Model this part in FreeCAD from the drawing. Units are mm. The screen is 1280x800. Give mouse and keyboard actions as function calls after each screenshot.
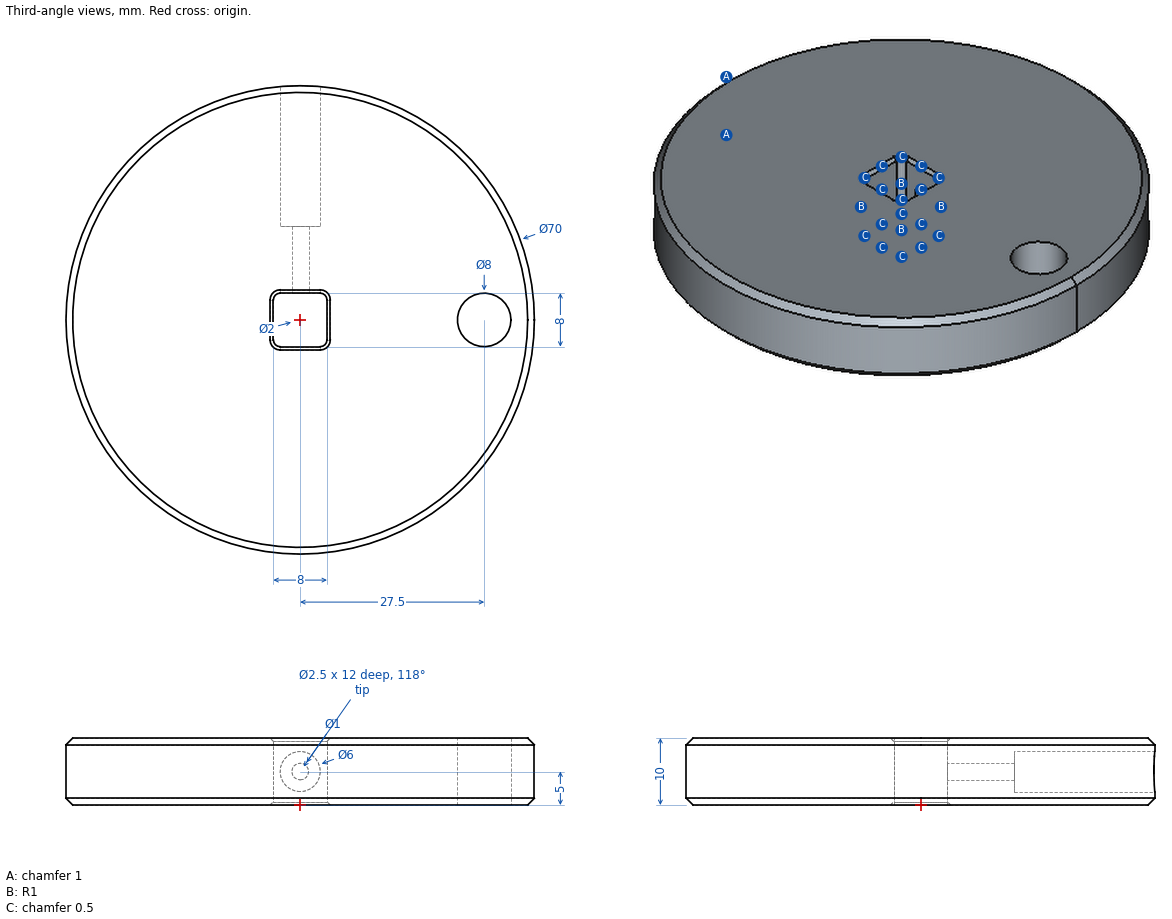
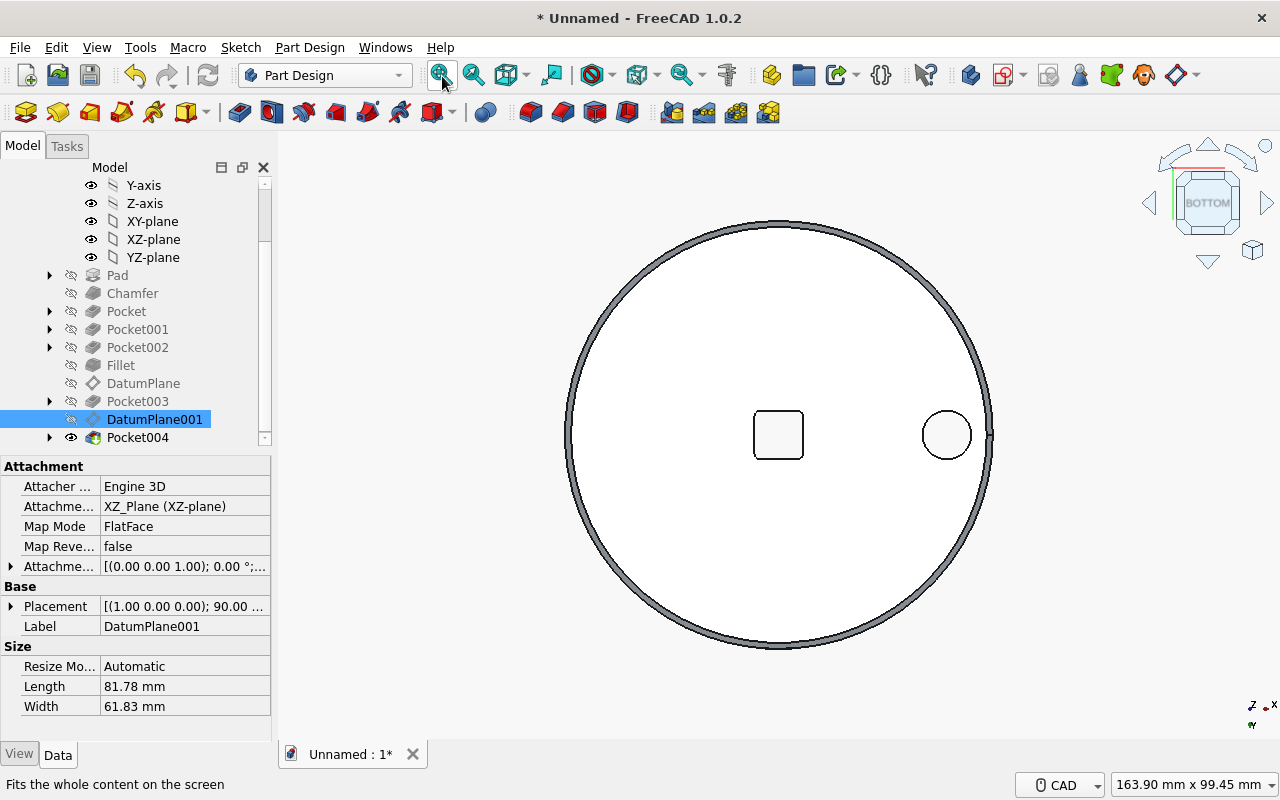
key(3)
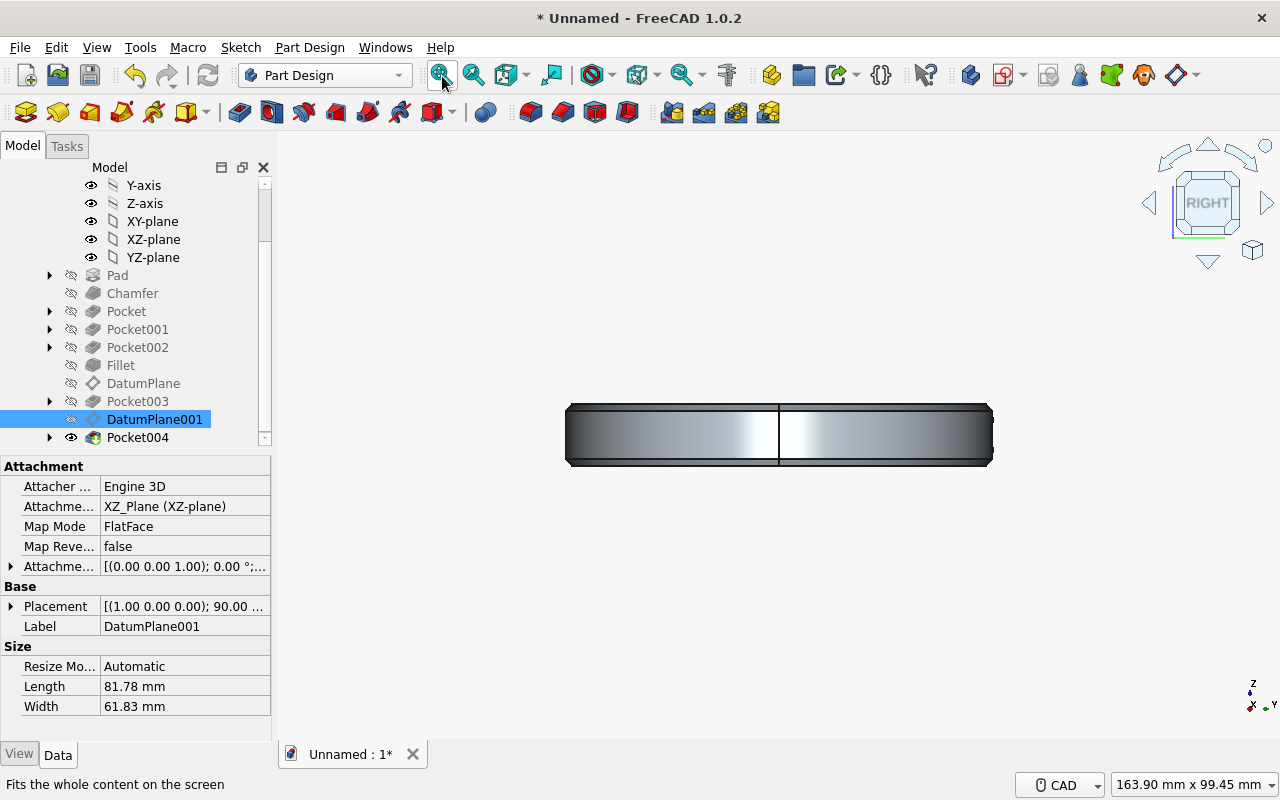
click(442, 76)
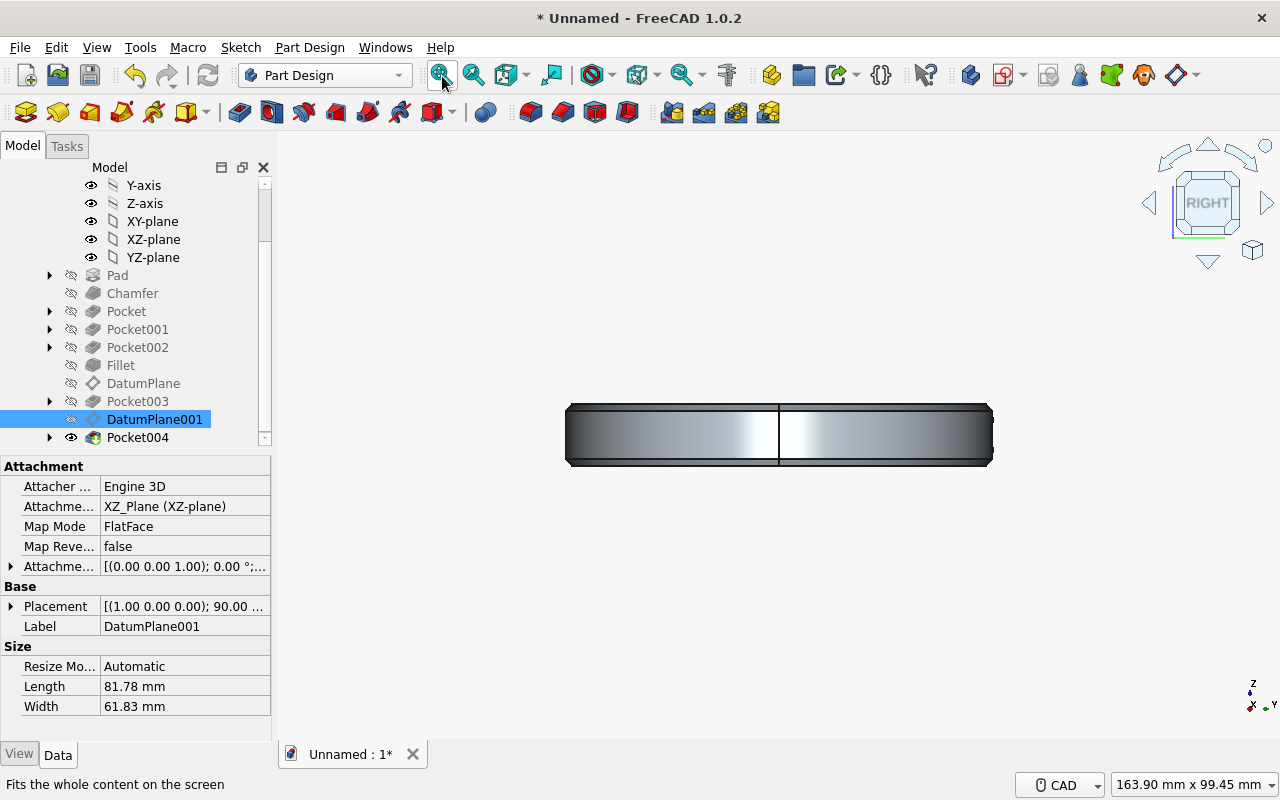
scroll(160, 307, down, 3)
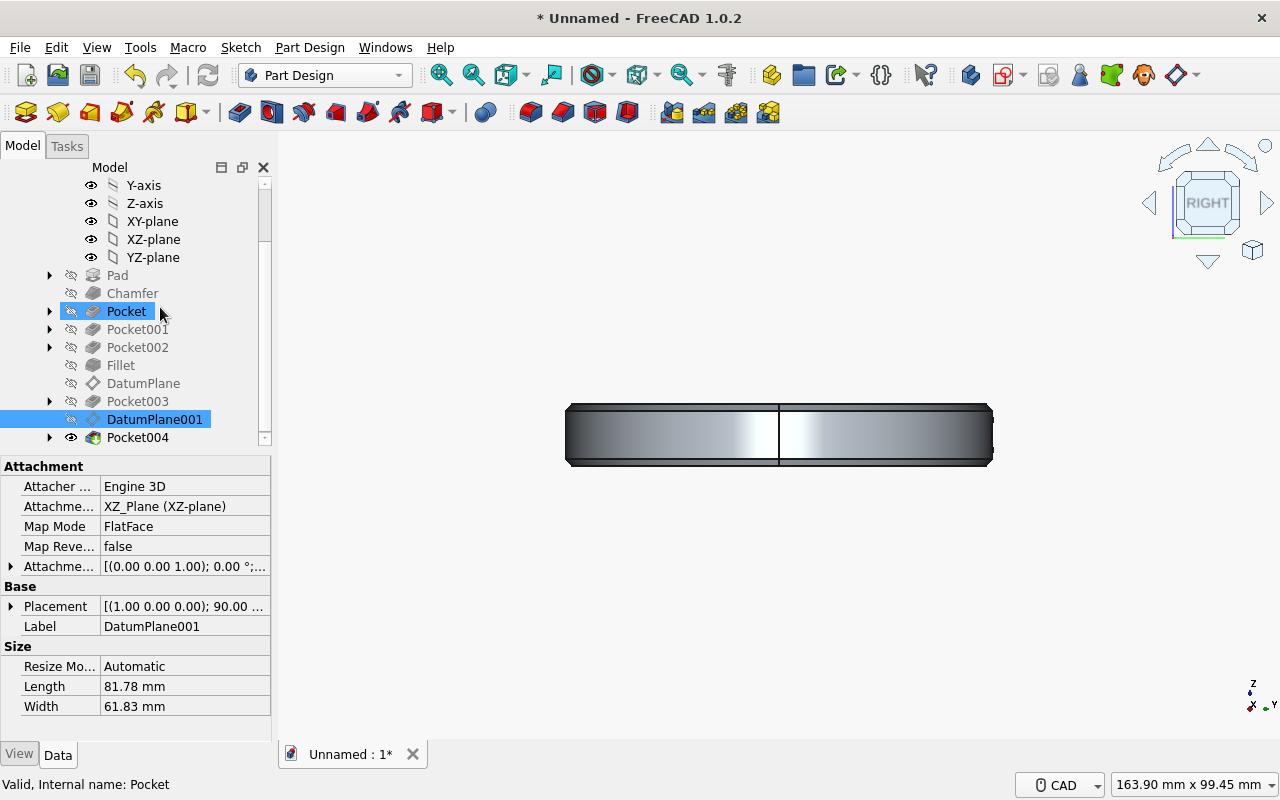
scroll(160, 307, up, 15)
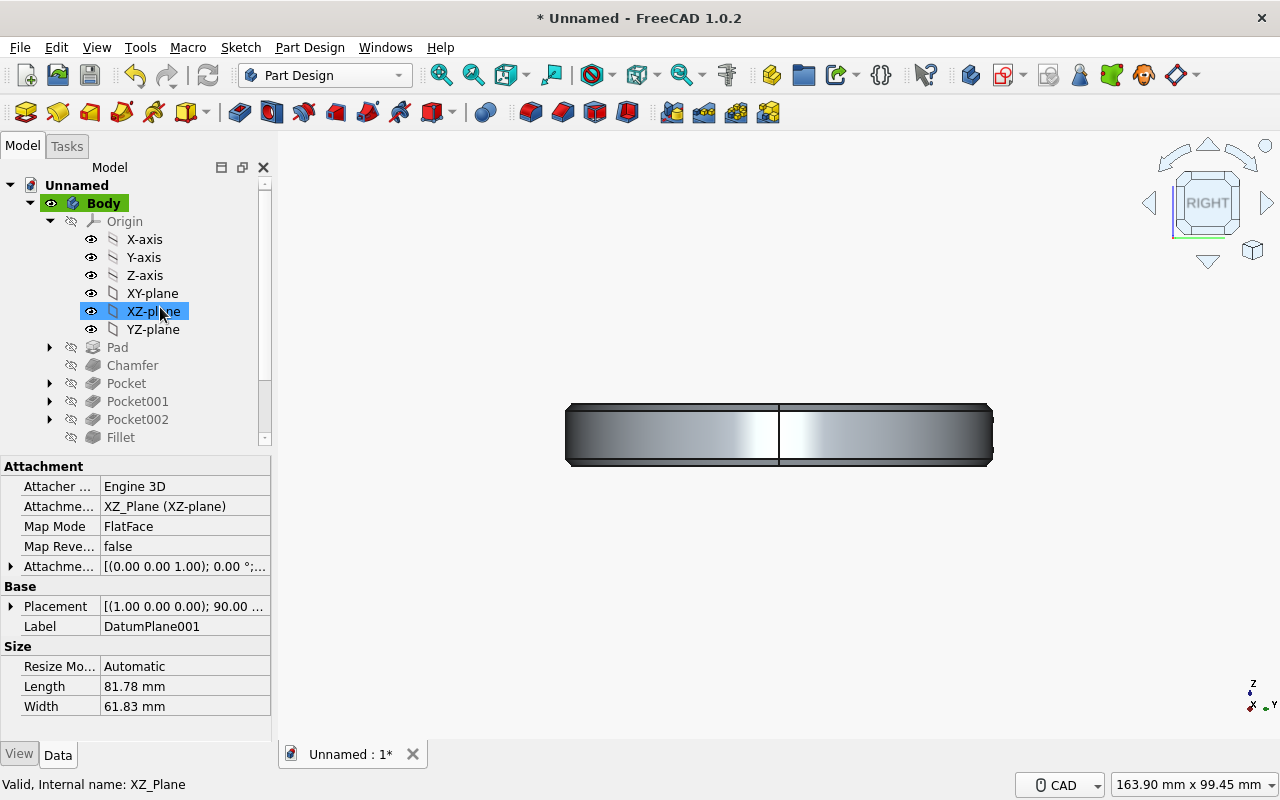
click(136, 311)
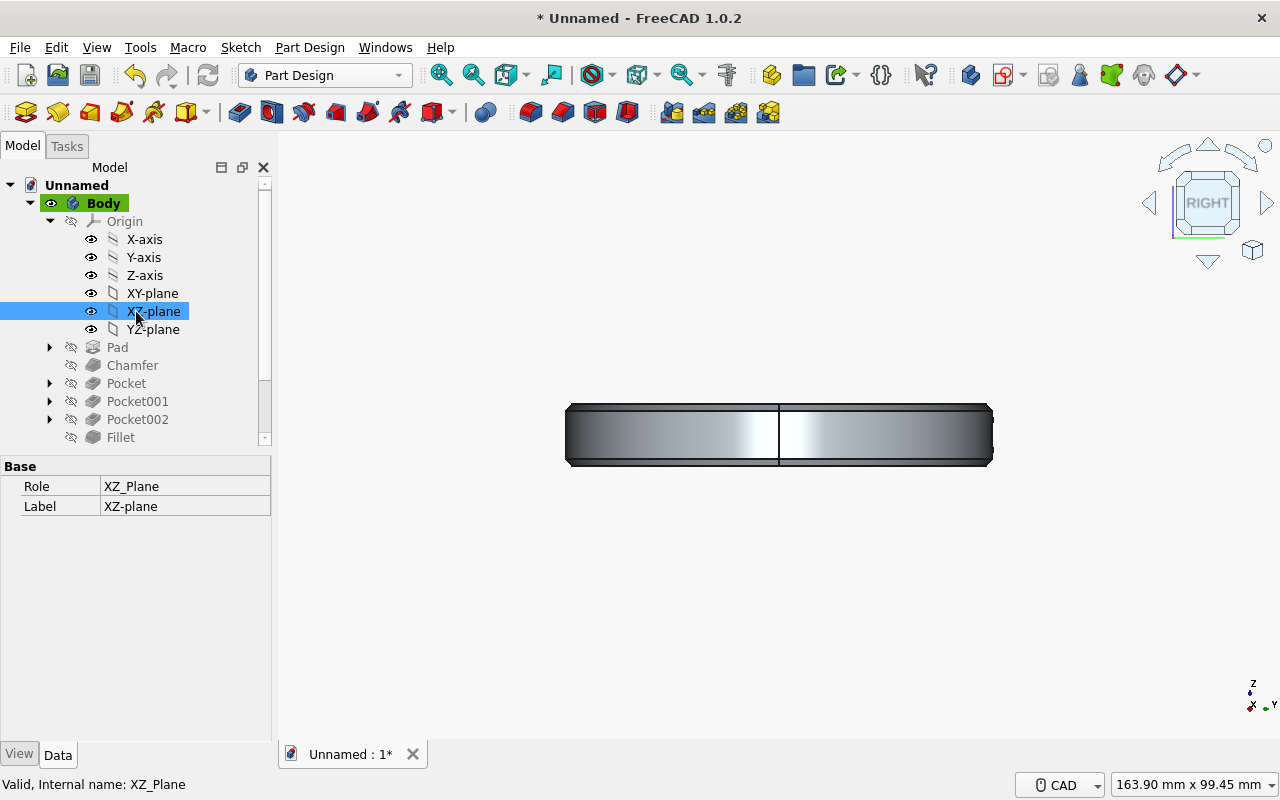
click(1176, 76)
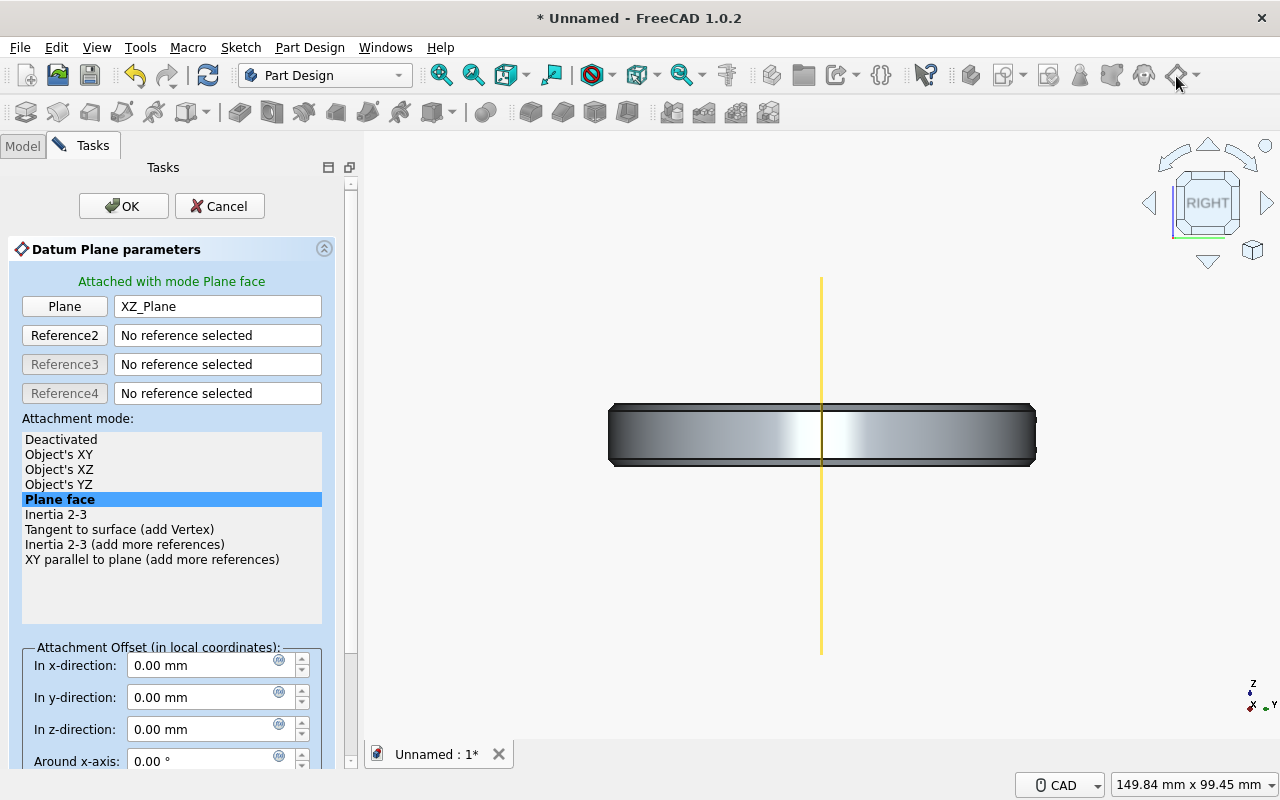
triple_click(210, 729)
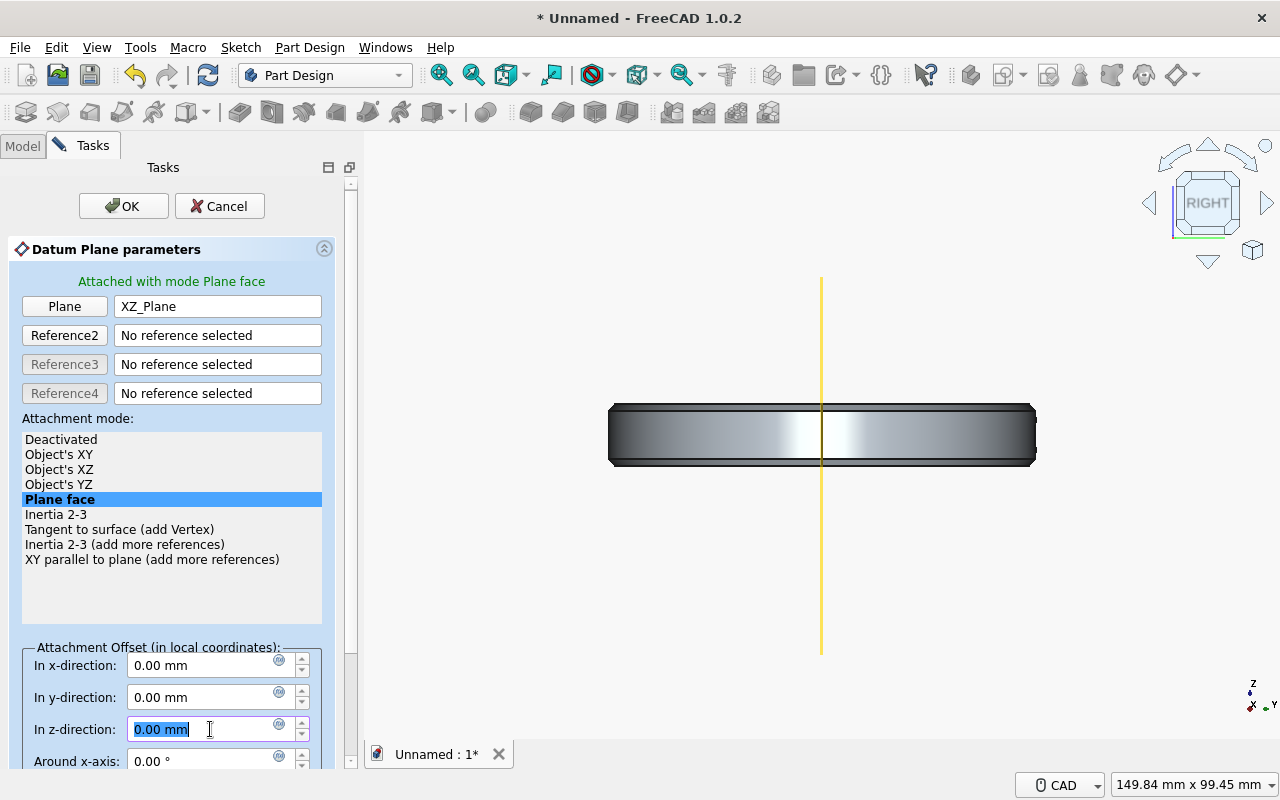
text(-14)
key(Tab)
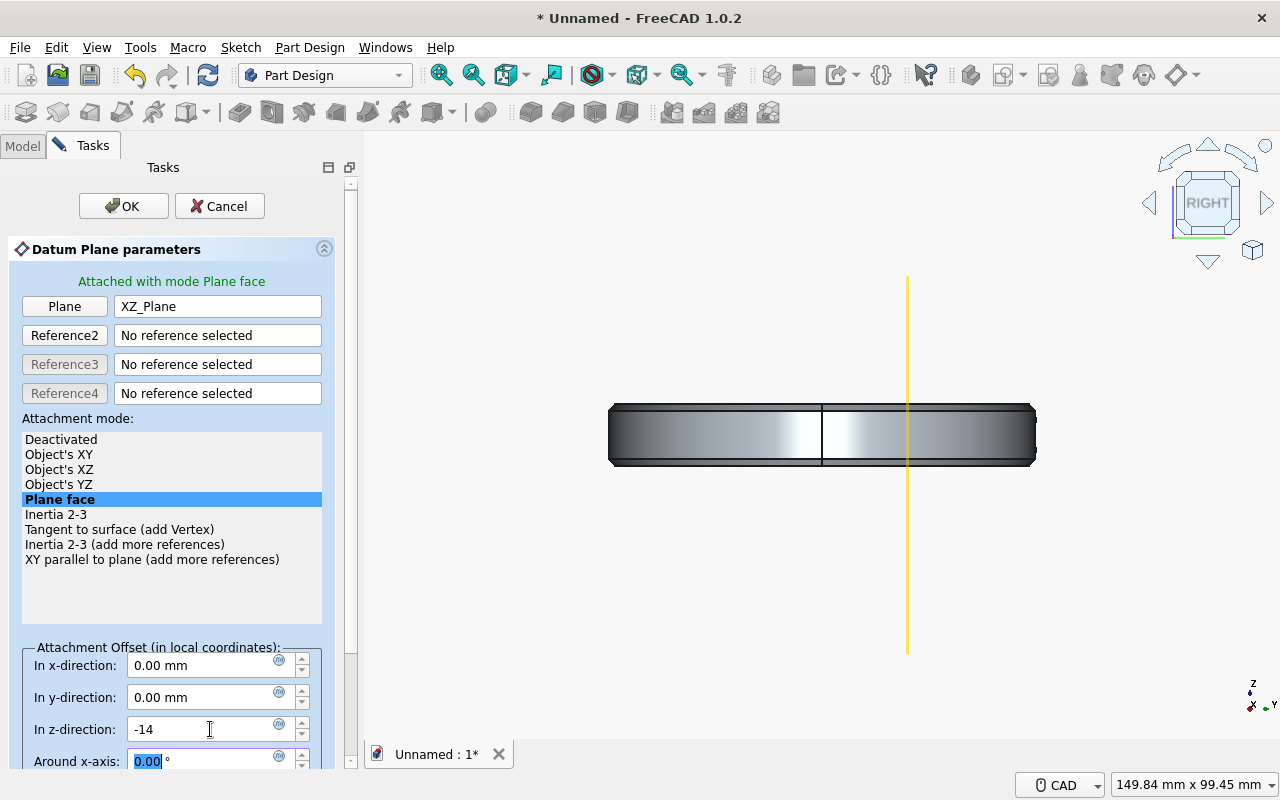
click(124, 206)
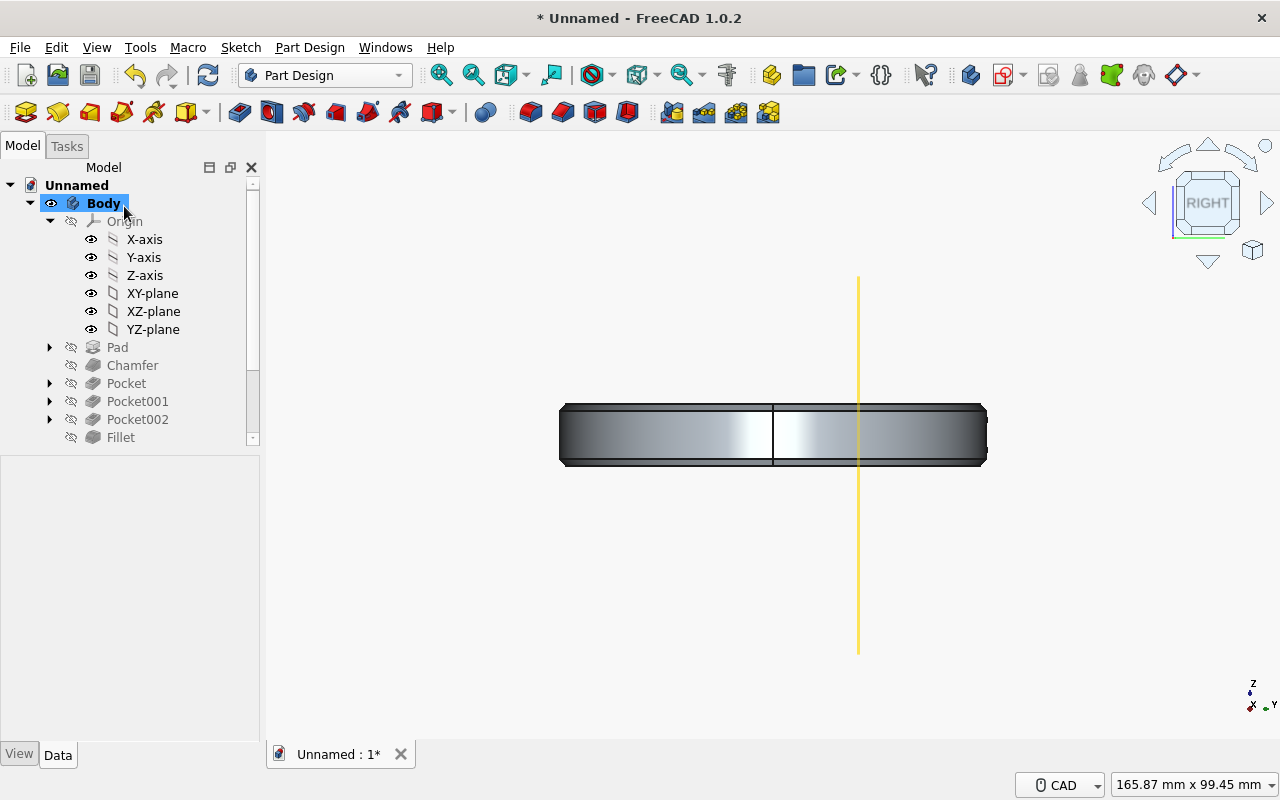
scroll(100, 307, down, 3)